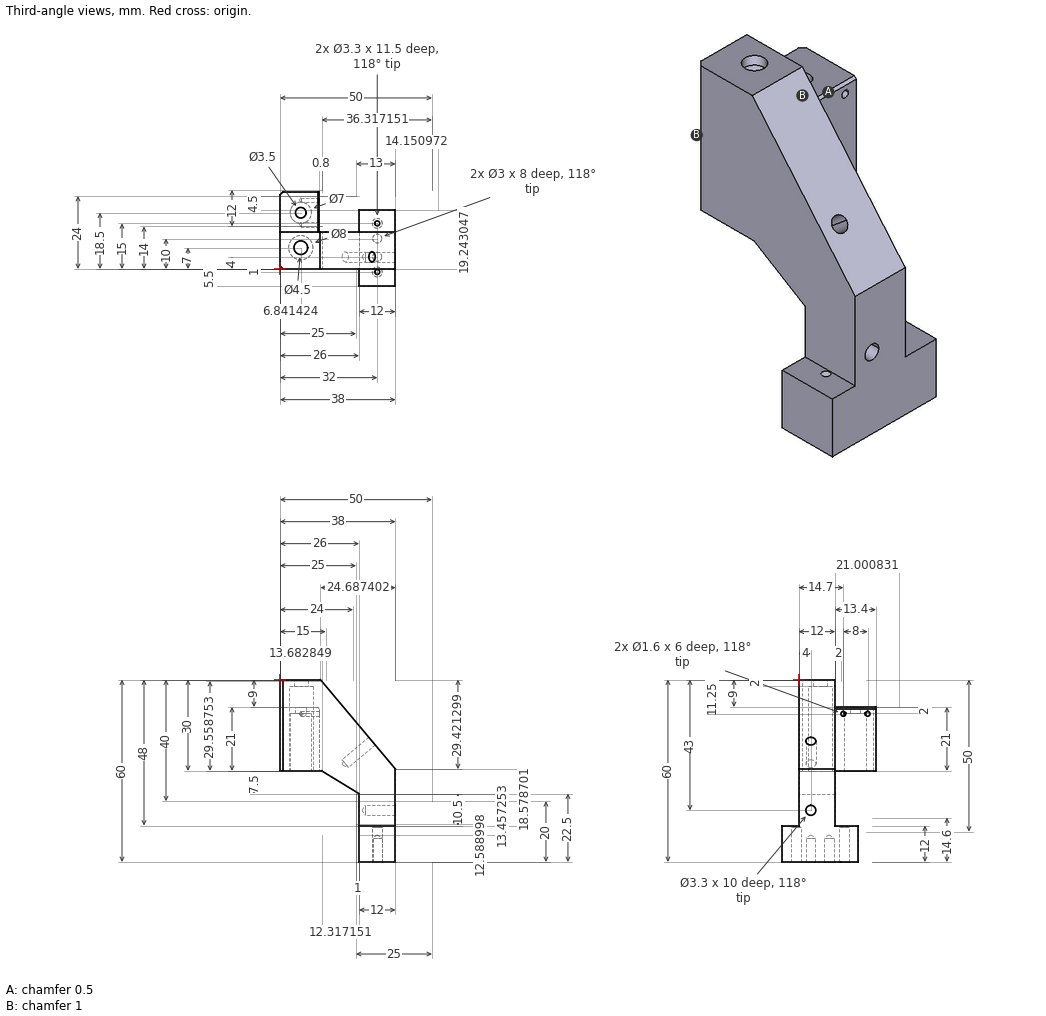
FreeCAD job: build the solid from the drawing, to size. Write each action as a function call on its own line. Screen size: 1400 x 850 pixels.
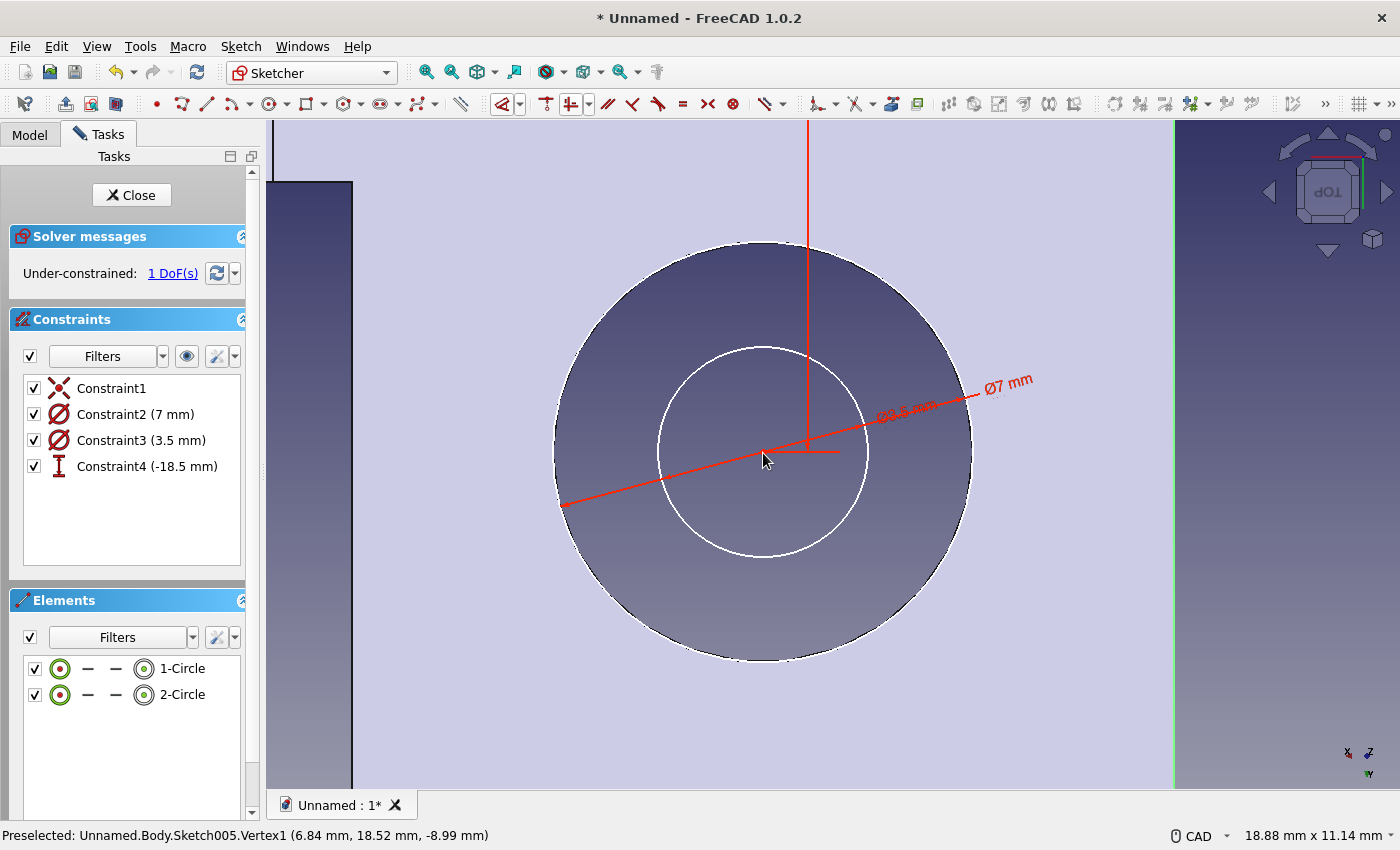
click(763, 452)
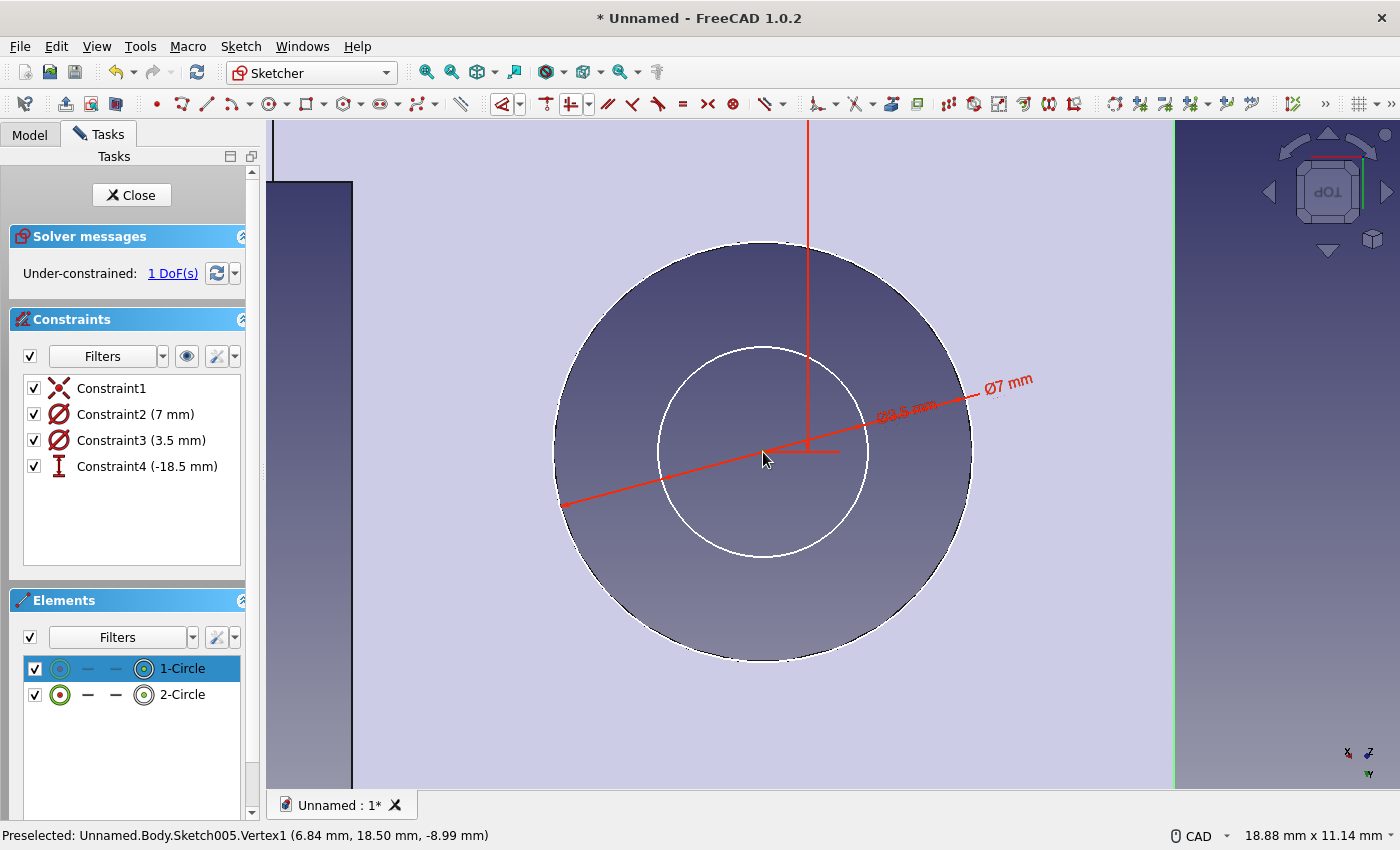
click(520, 104)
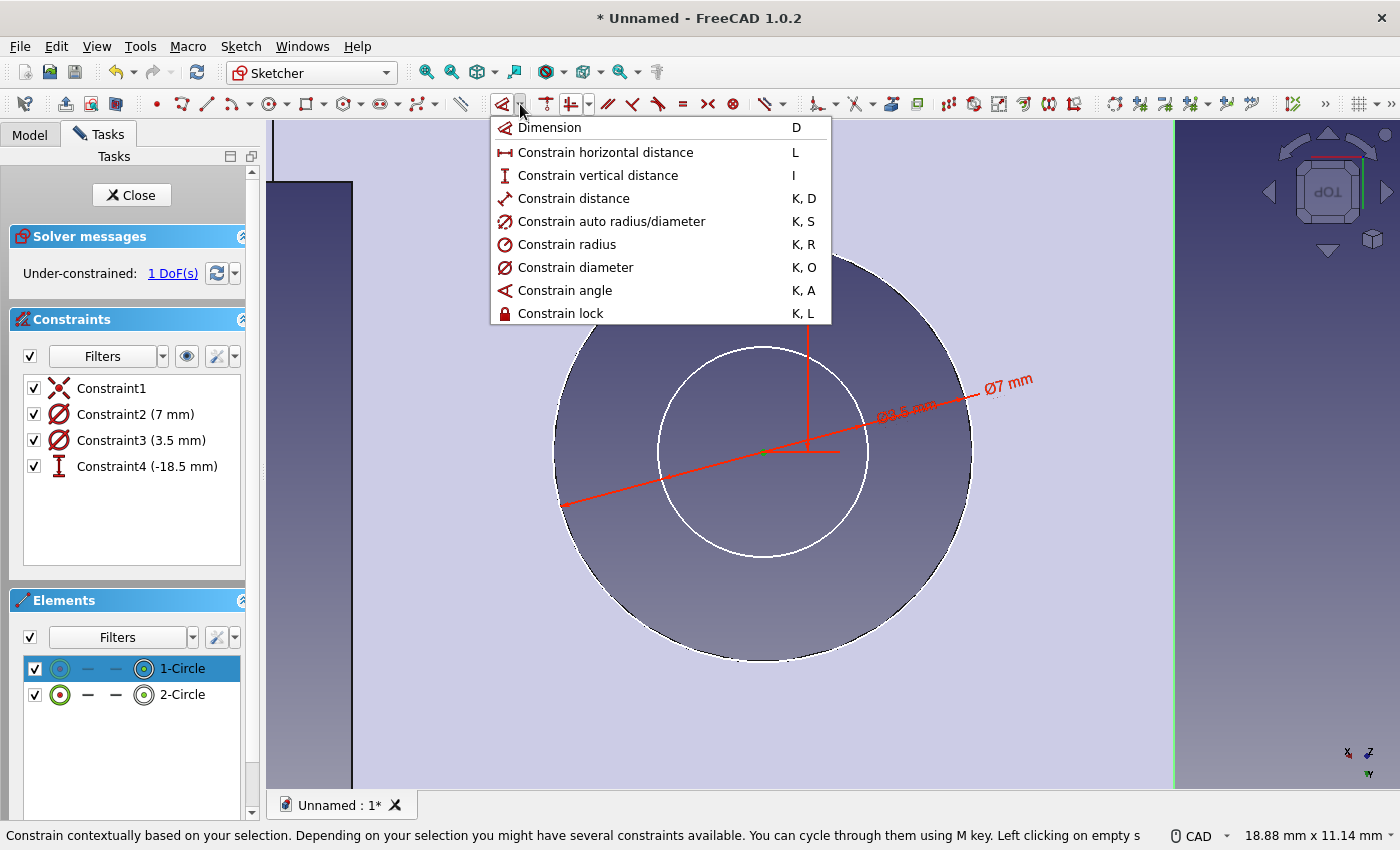
click(661, 152)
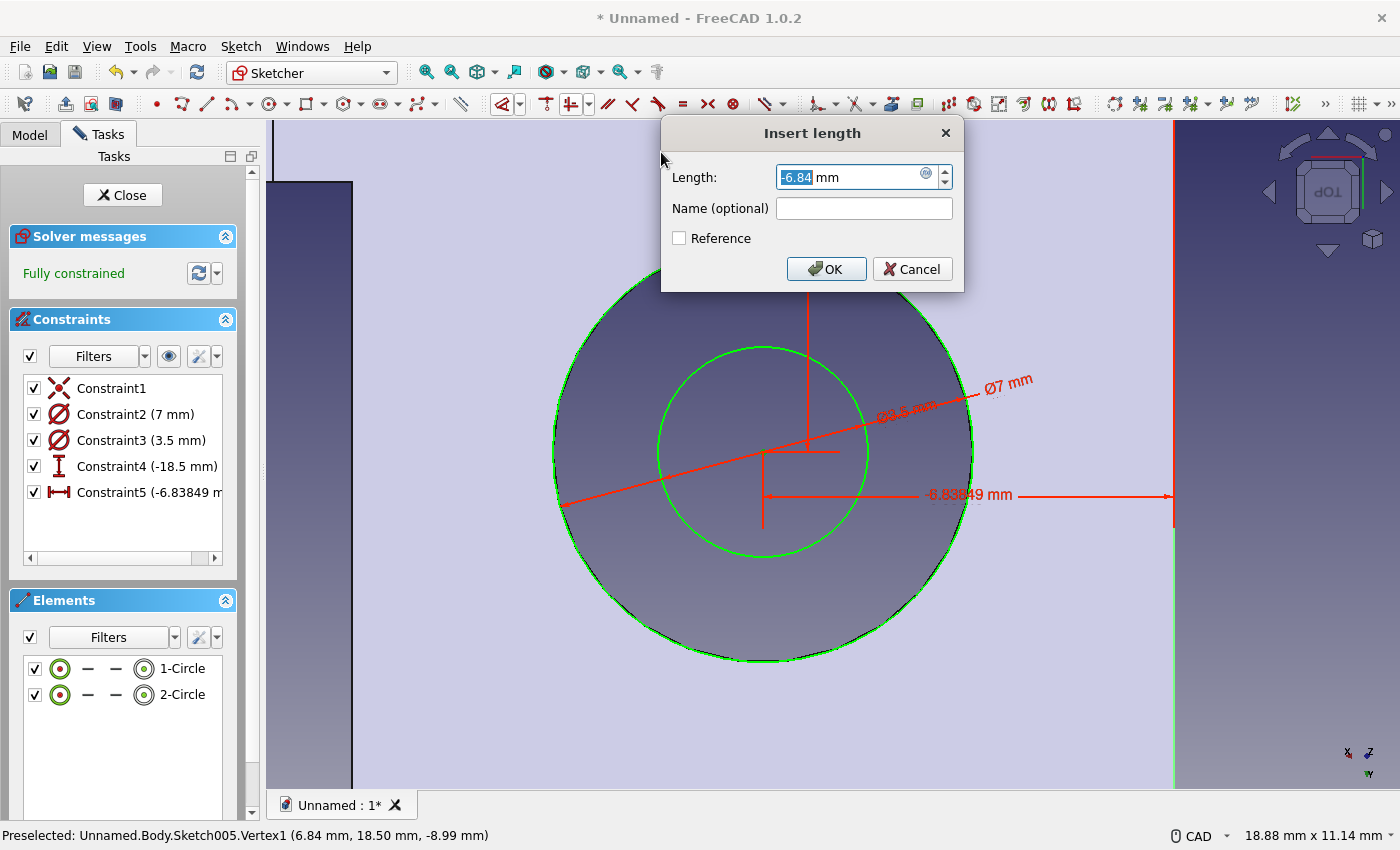
text(-6.841424)
key(Return)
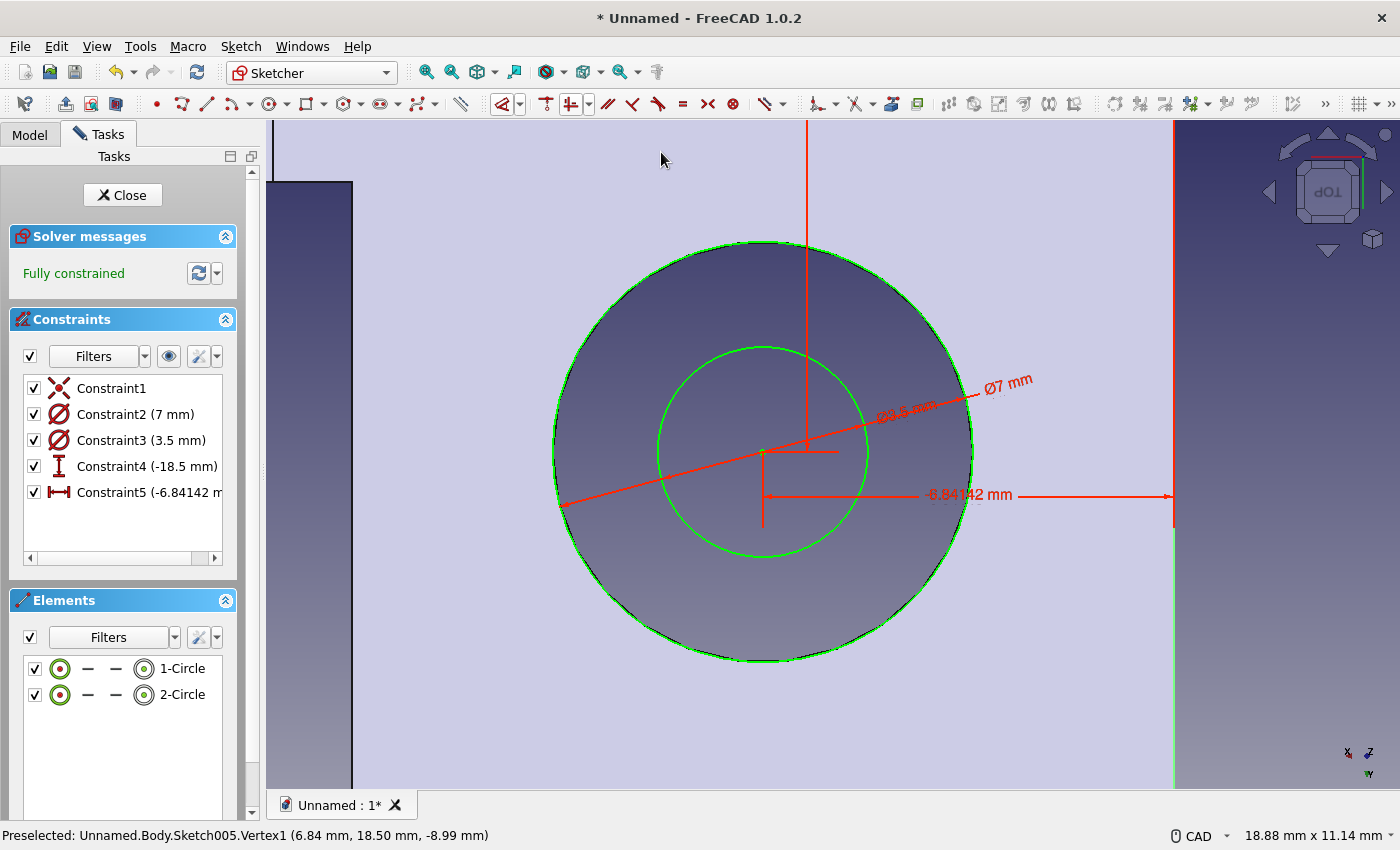
click(123, 195)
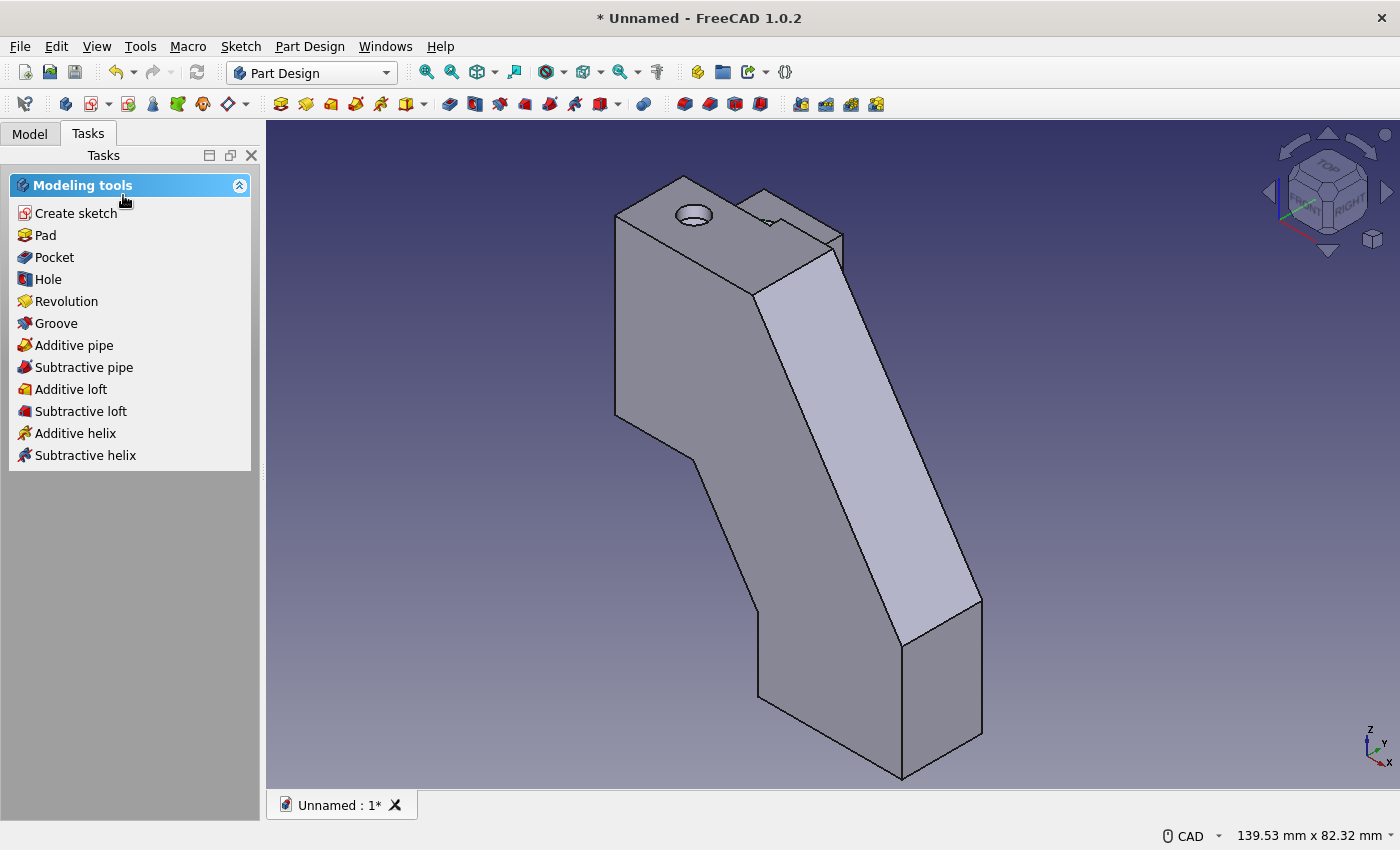
click(281, 104)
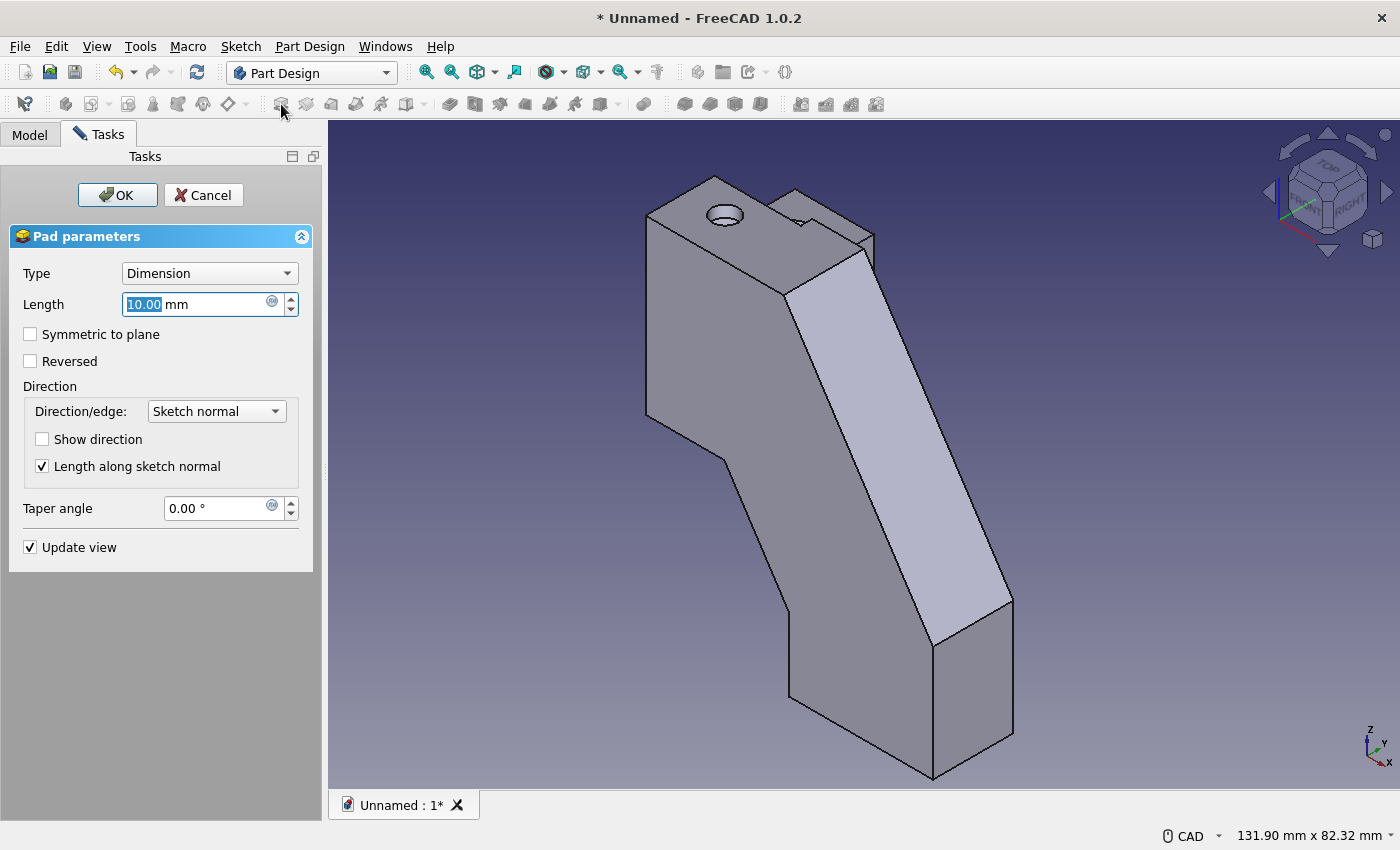
text(2)
key(Tab)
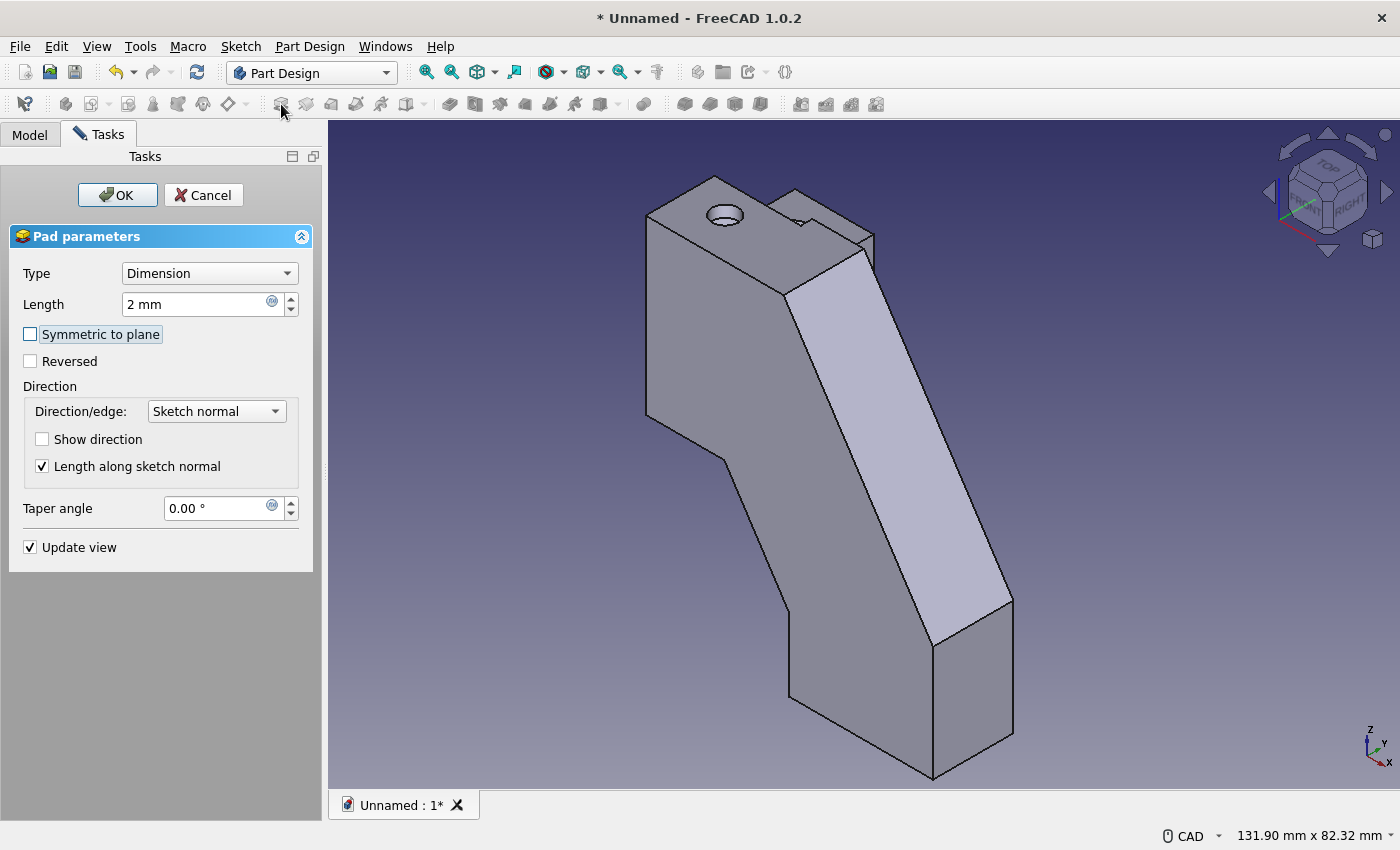
click(31, 361)